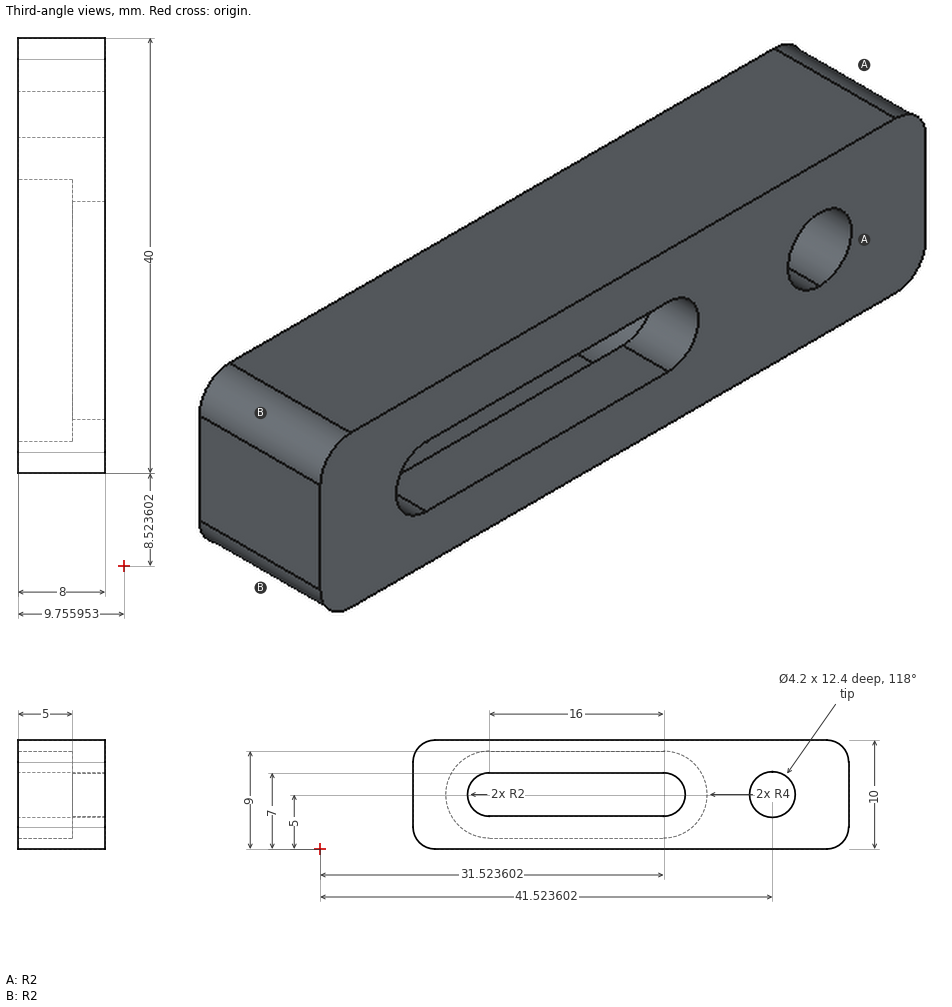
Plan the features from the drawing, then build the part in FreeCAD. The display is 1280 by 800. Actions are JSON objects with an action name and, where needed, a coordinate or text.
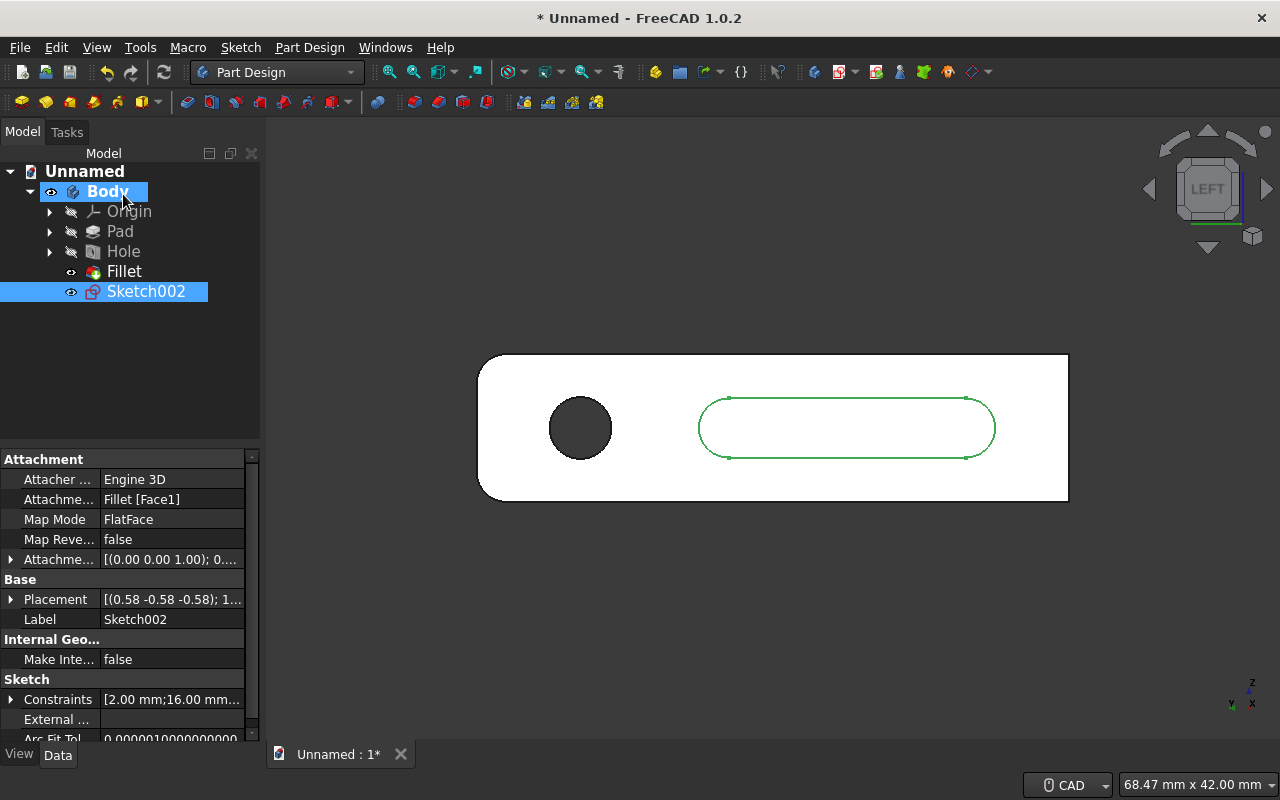
{"action": "left_click", "coordinate": [188, 102]}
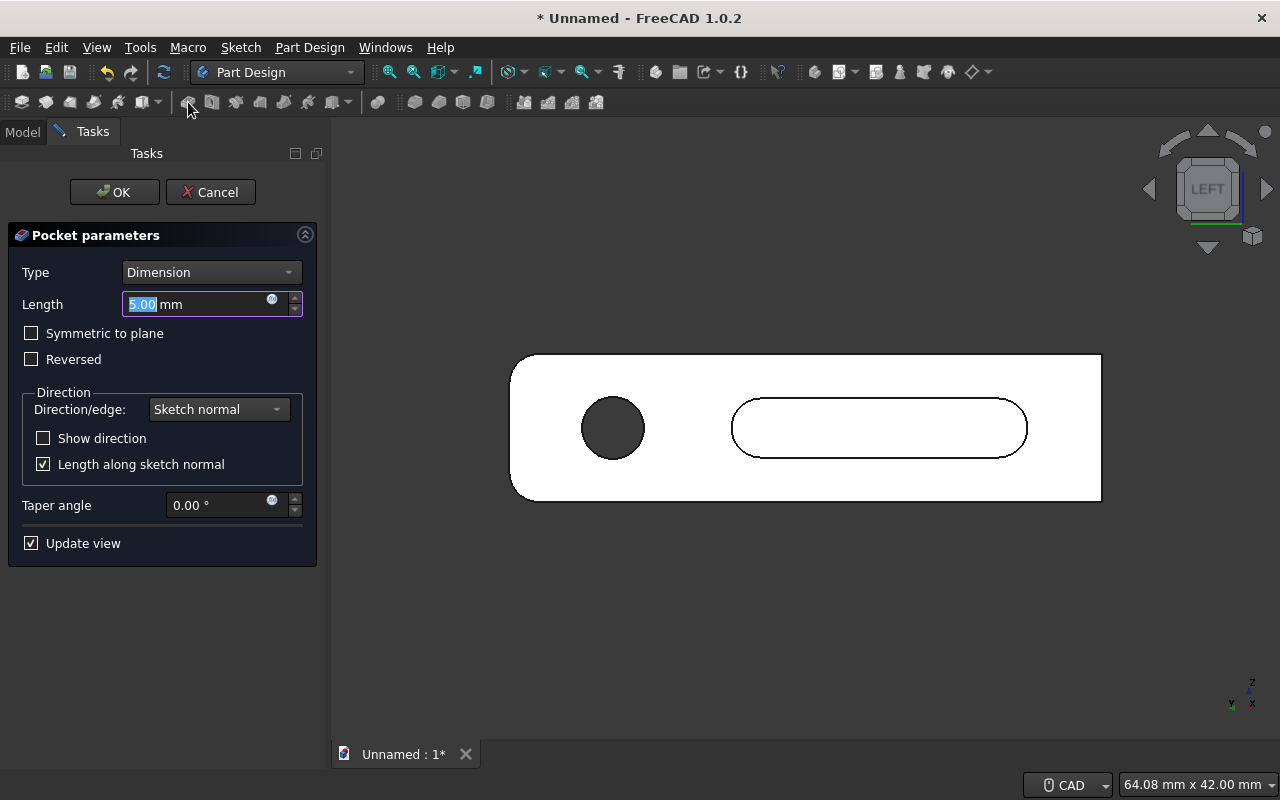
{"action": "left_click", "coordinate": [212, 272]}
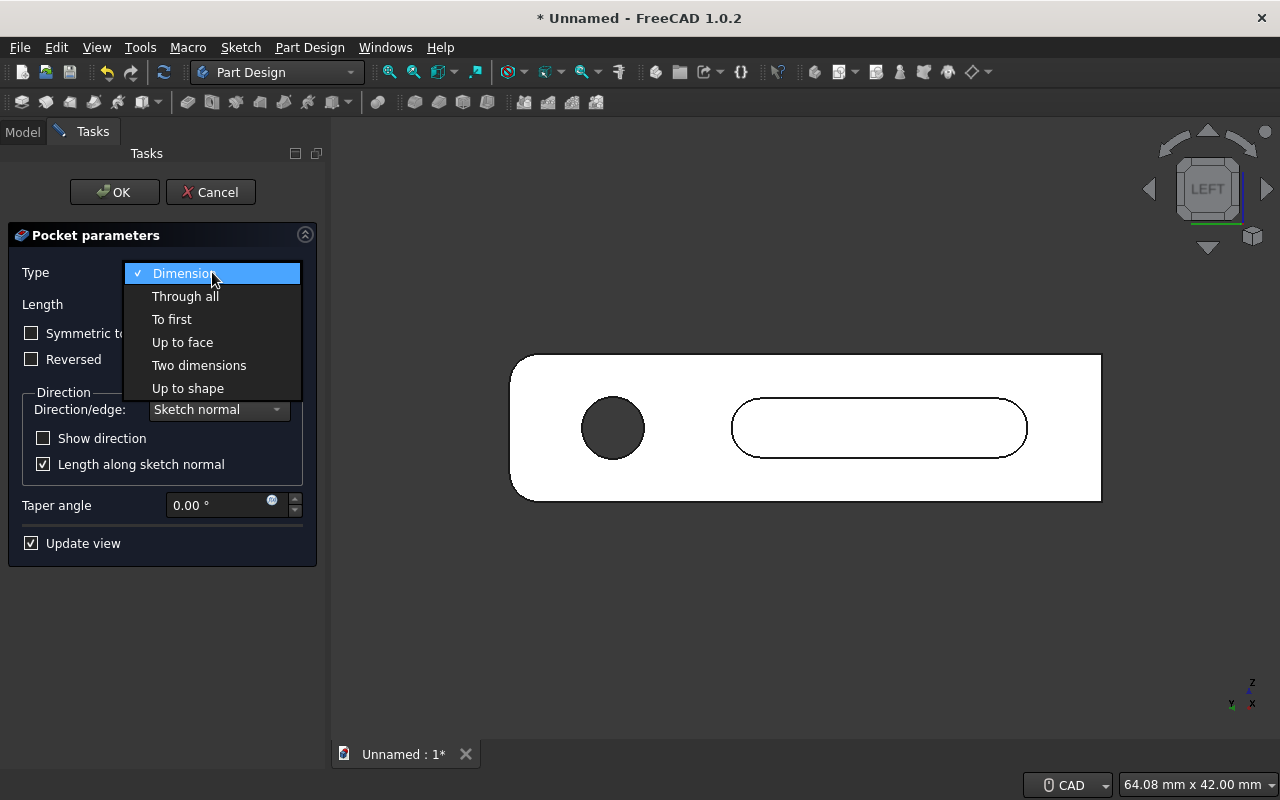
{"action": "left_click", "coordinate": [212, 296]}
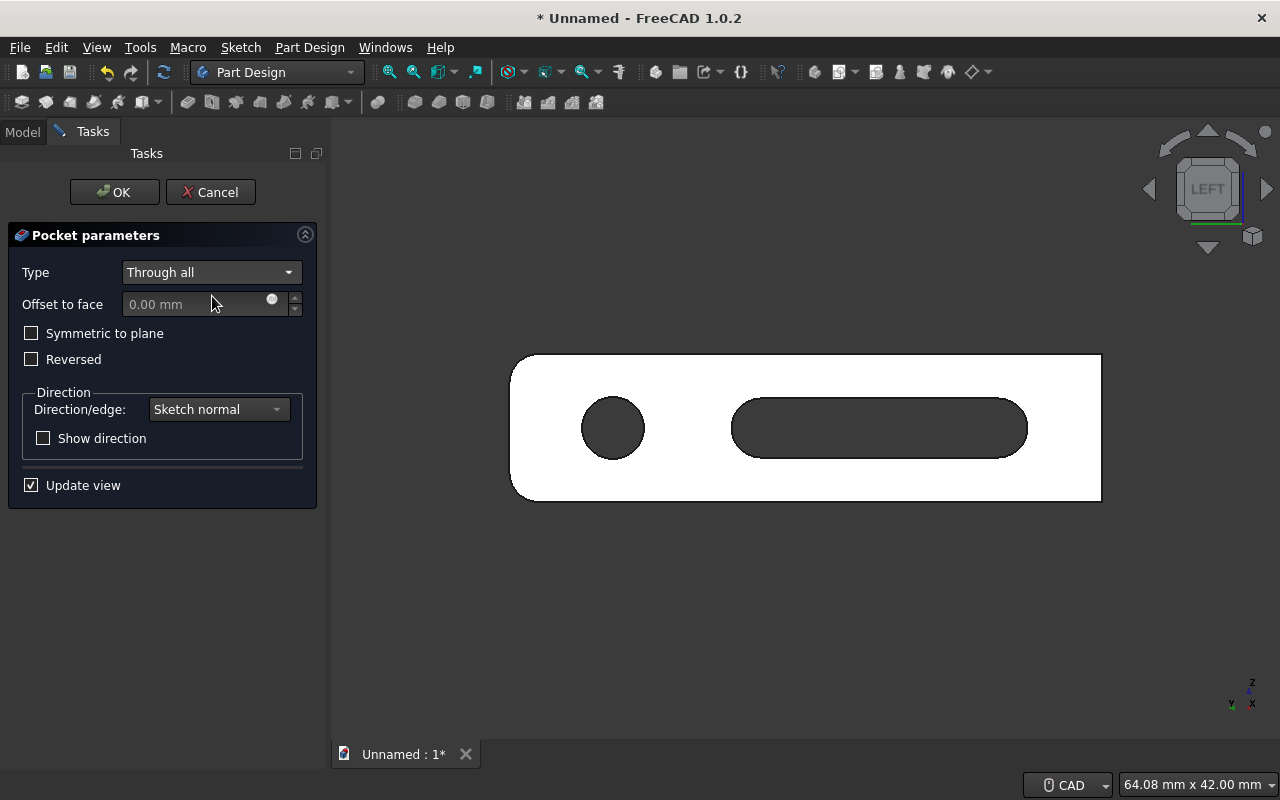
{"action": "left_click", "coordinate": [115, 192]}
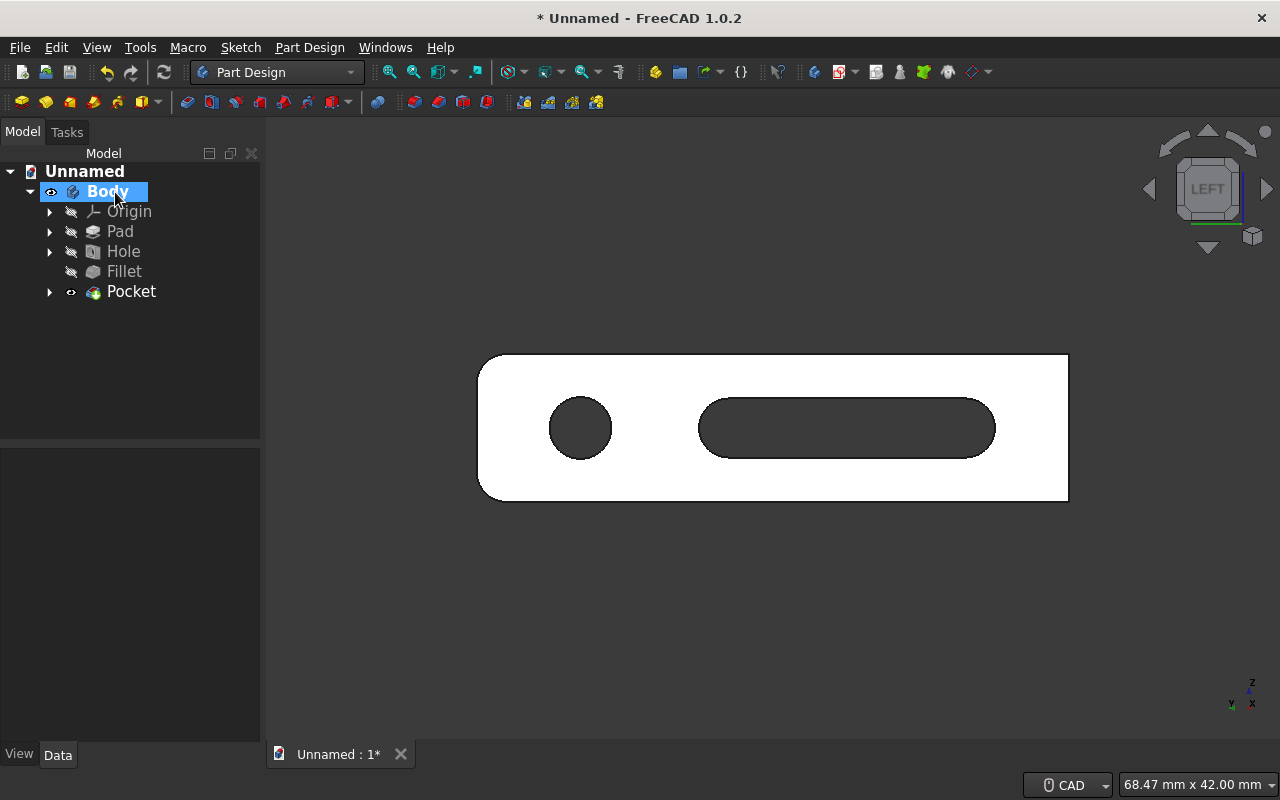
{"action": "left_click", "coordinate": [1027, 406]}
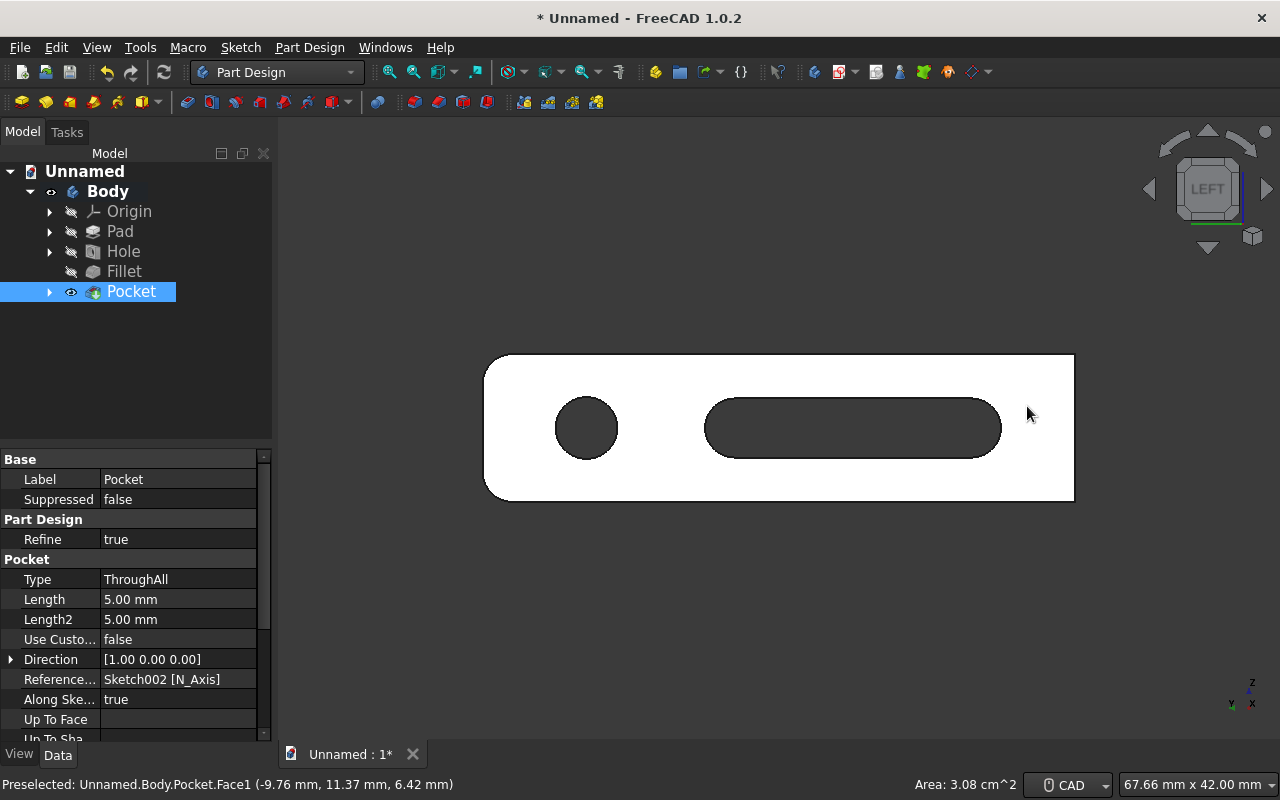
{"action": "left_click", "coordinate": [840, 72]}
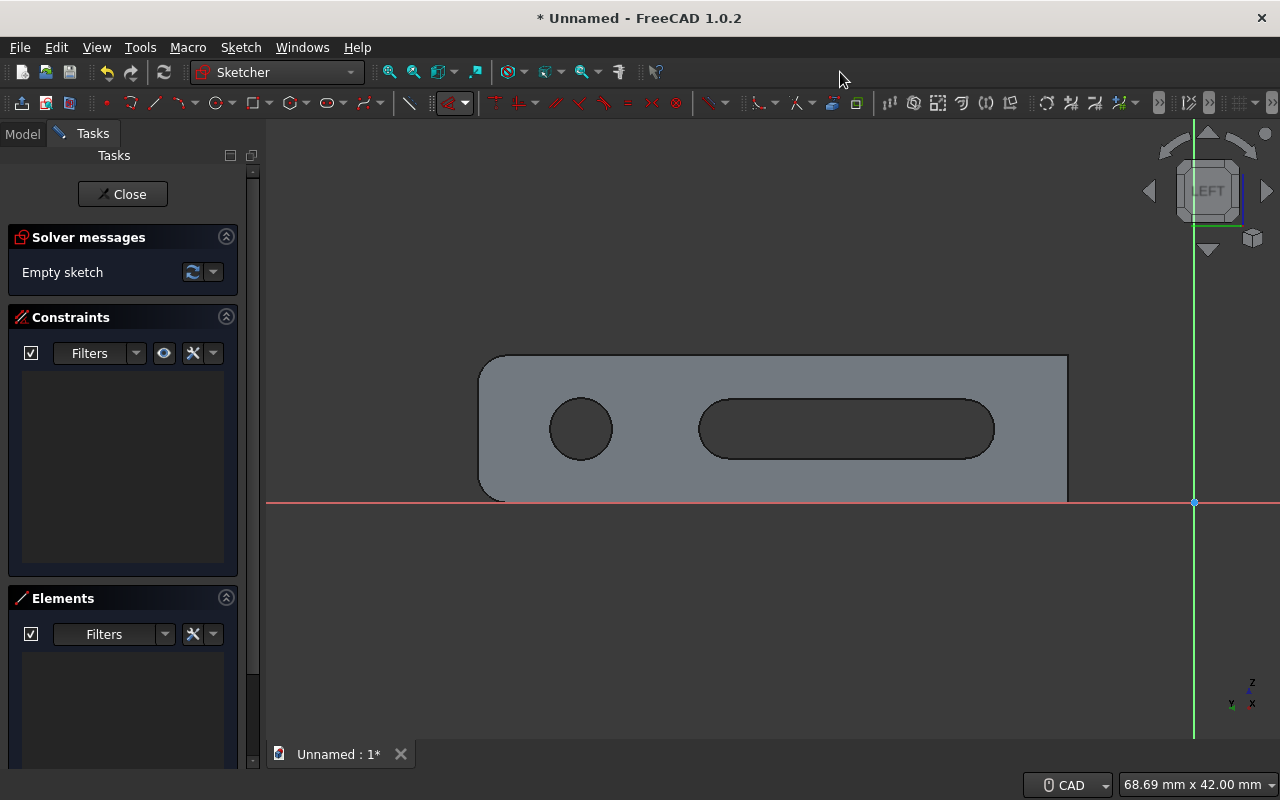
{"action": "scroll", "coordinate": [294, 396], "scroll_direction": "down", "scroll_amount": 1}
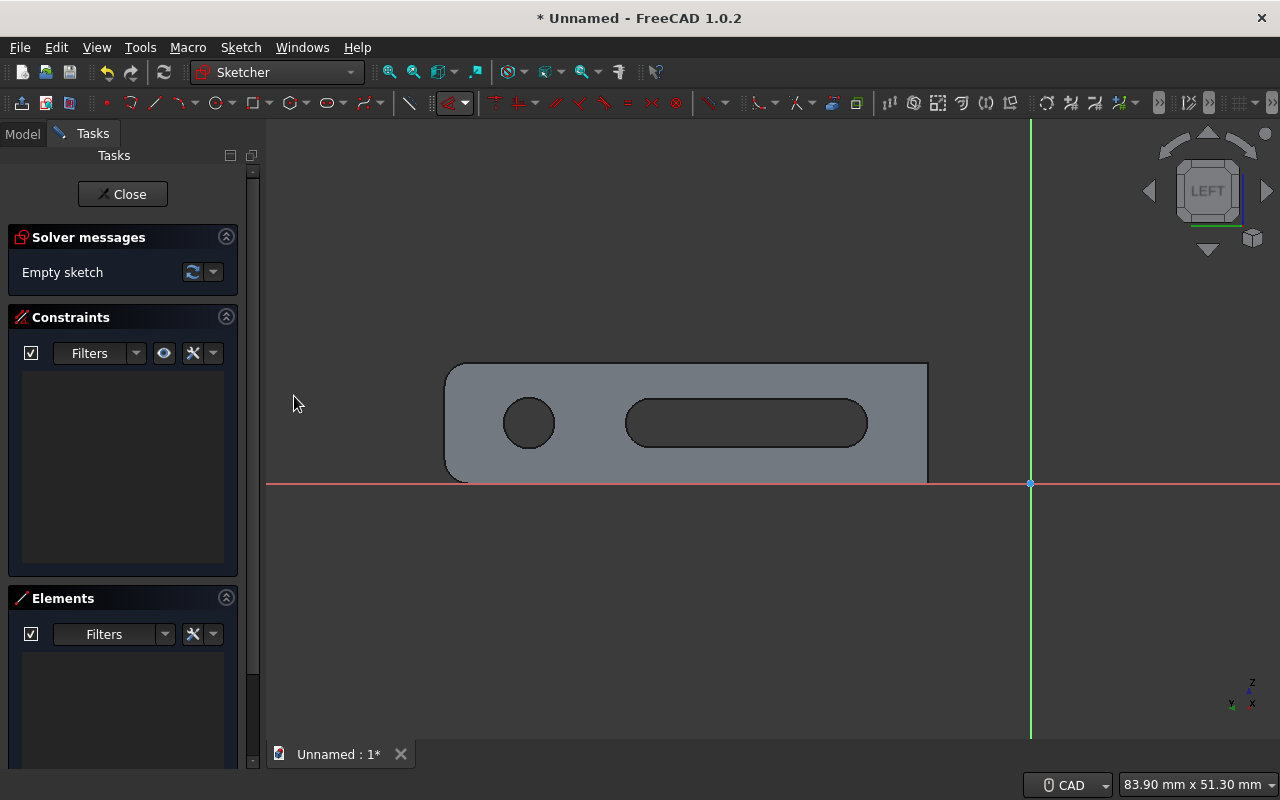
{"action": "left_click", "coordinate": [328, 104]}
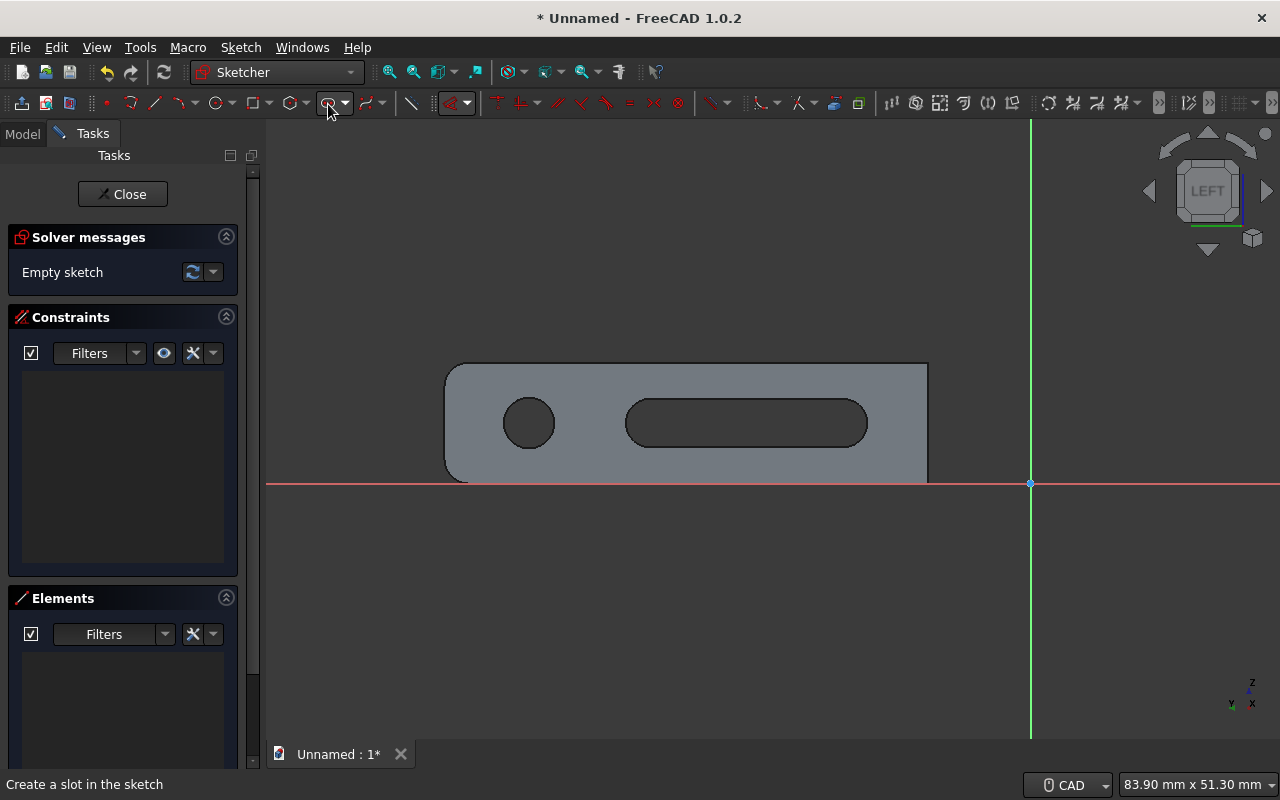
{"action": "left_click", "coordinate": [650, 423]}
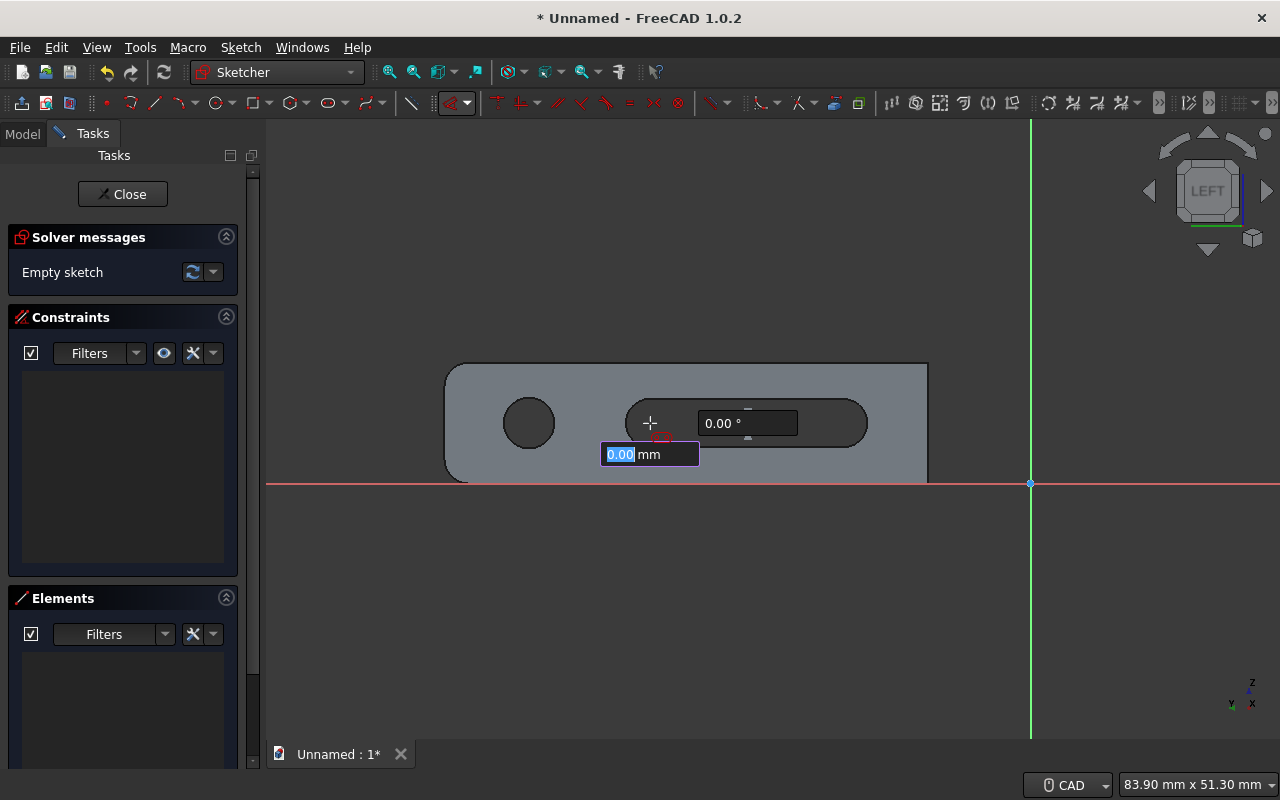
{"action": "left_click", "coordinate": [843, 423]}